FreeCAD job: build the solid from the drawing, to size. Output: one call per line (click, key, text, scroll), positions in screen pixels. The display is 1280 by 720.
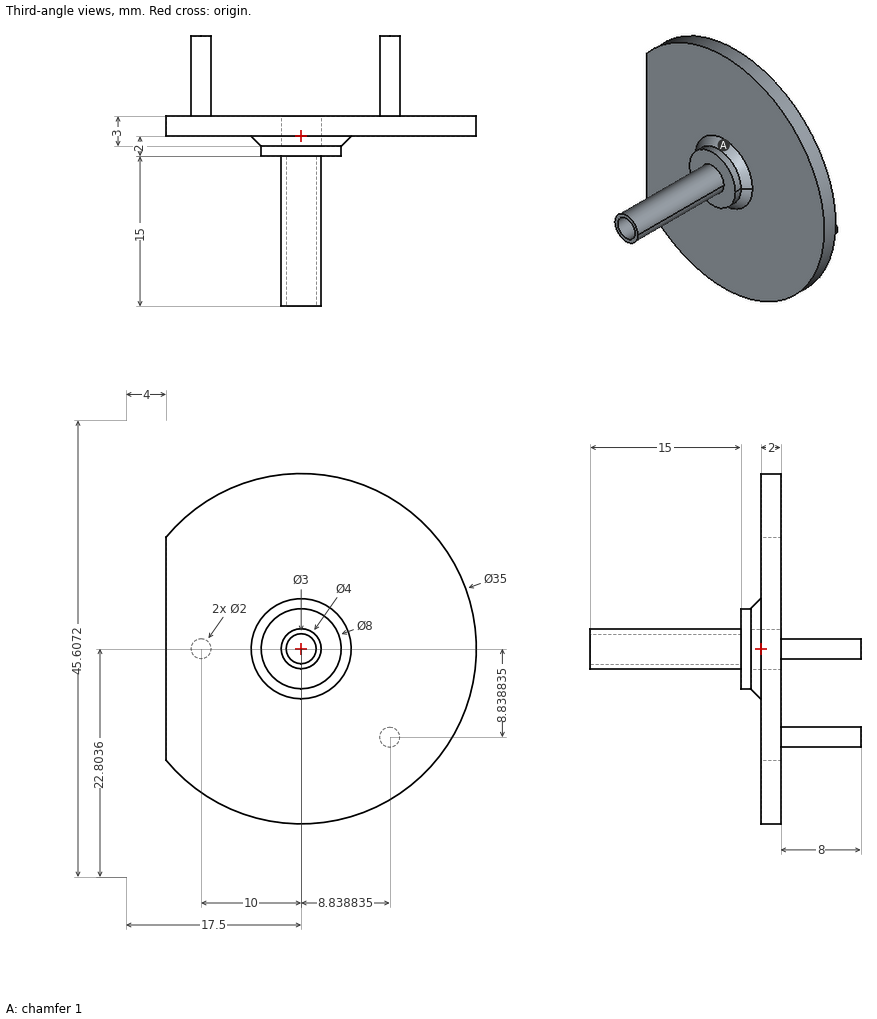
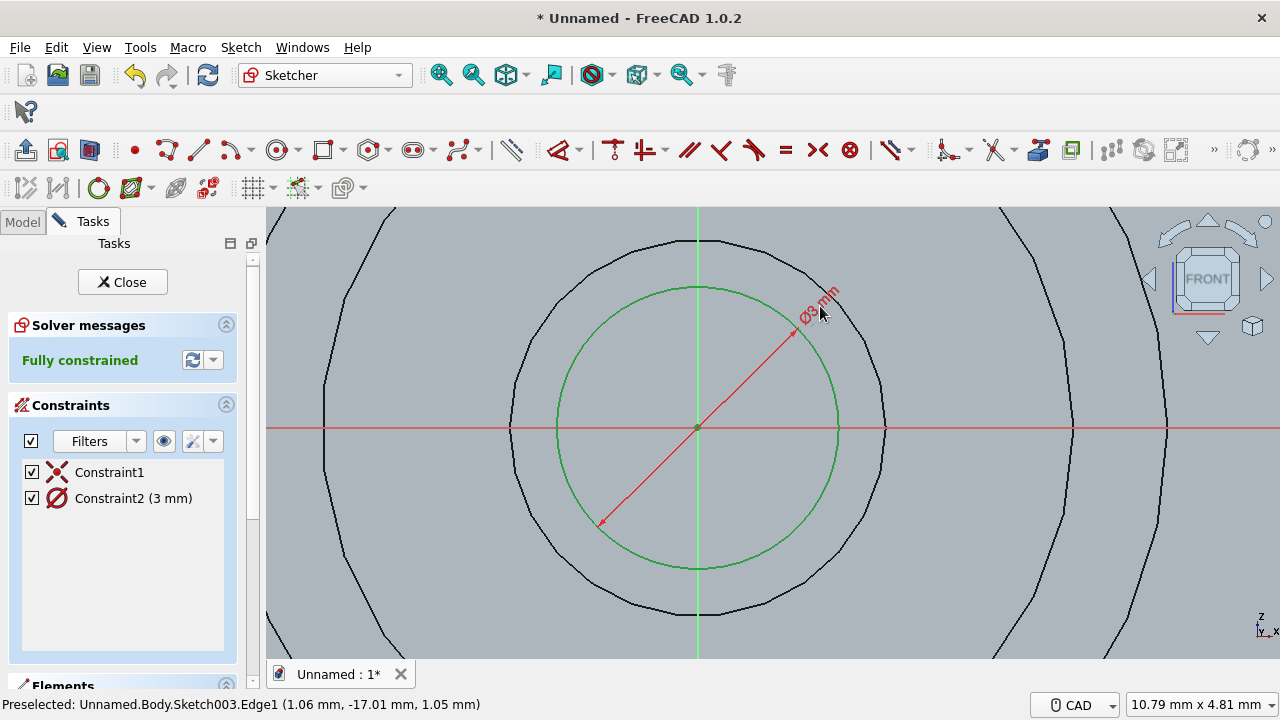
click(123, 282)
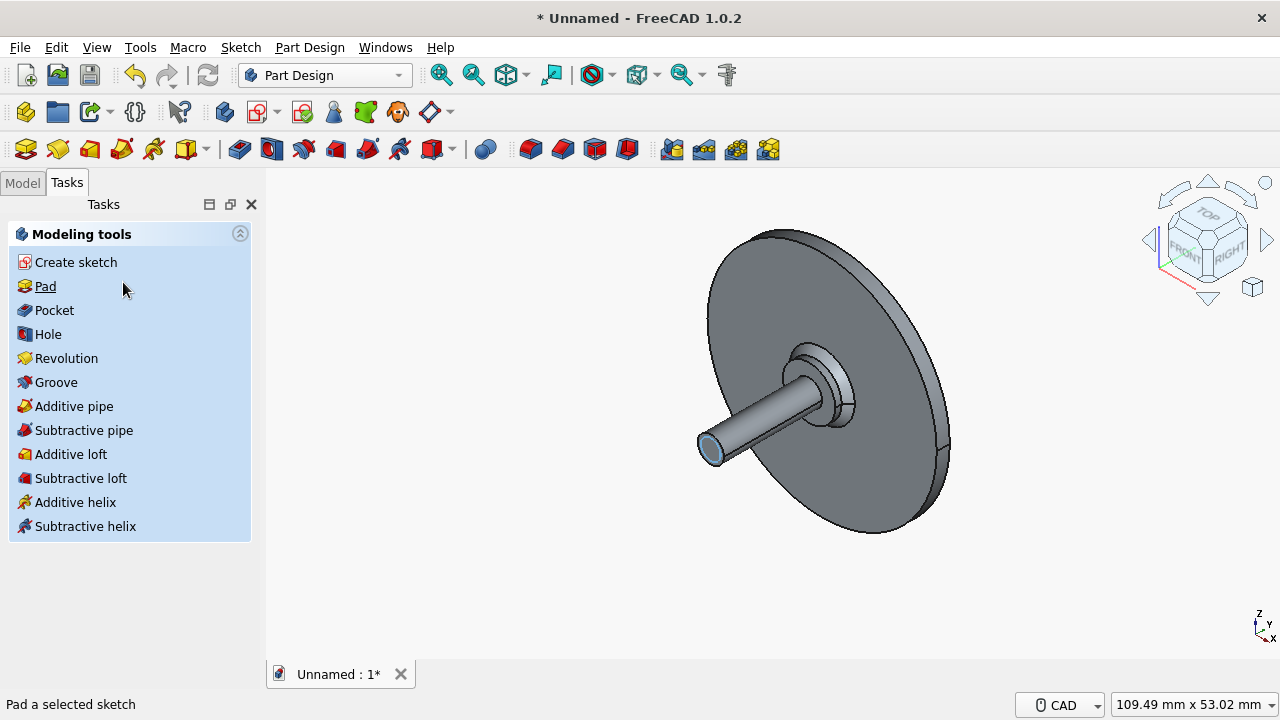
click(240, 150)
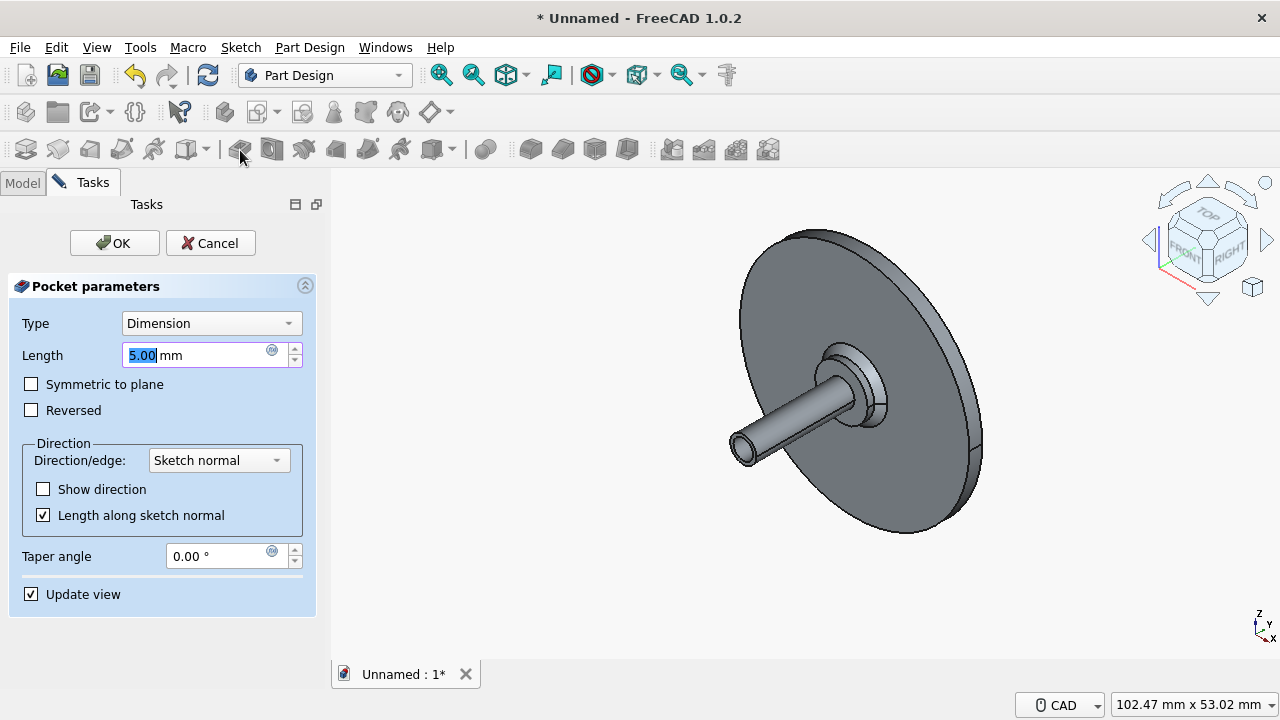
text(15)
key(Tab)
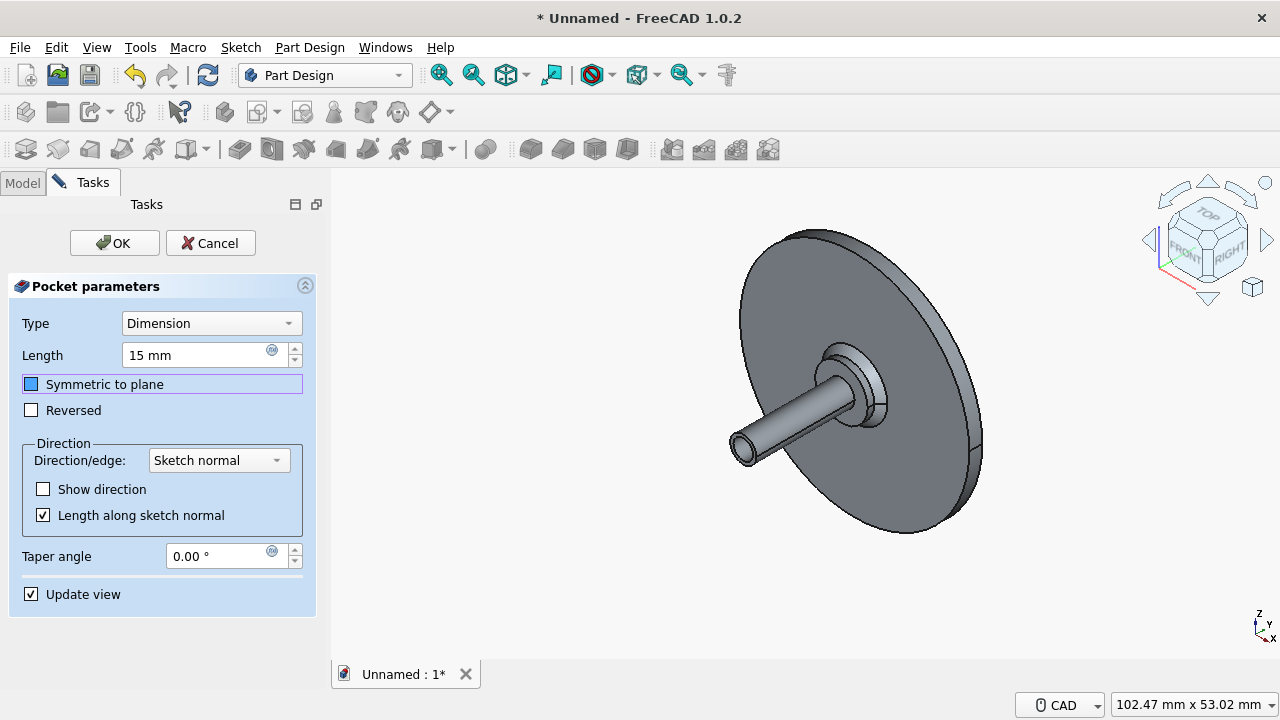
click(115, 243)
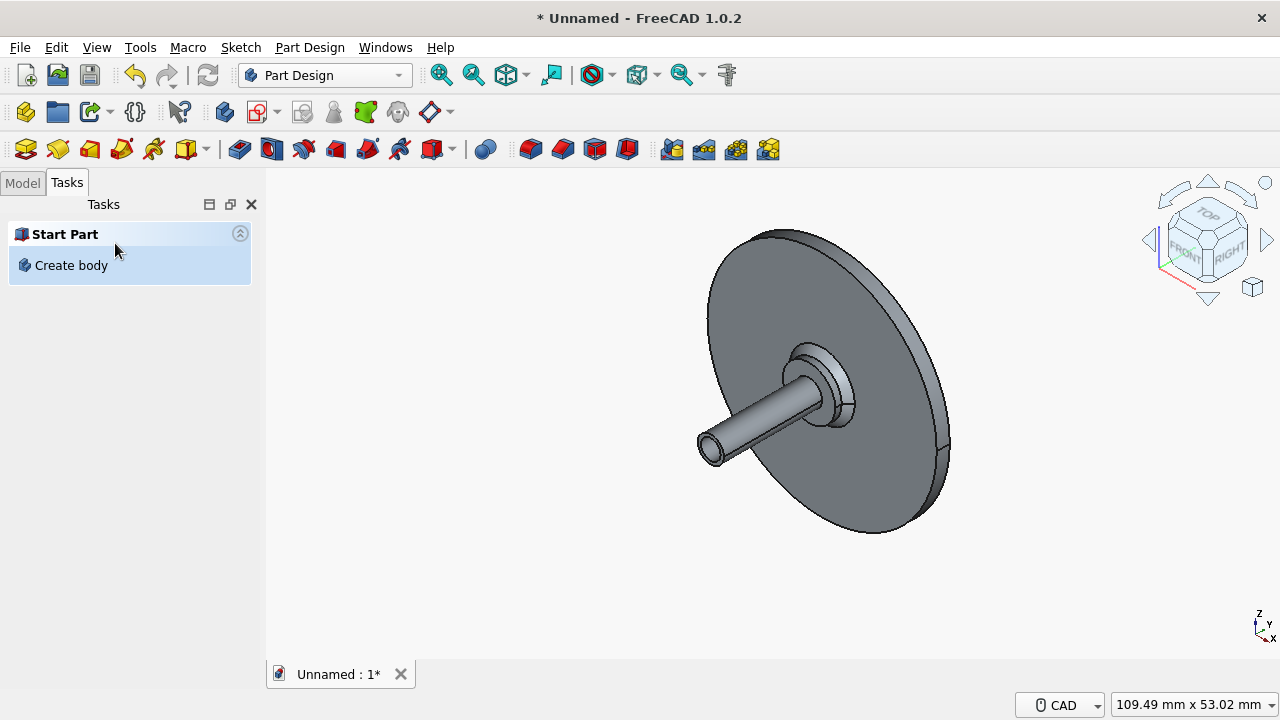
key(4)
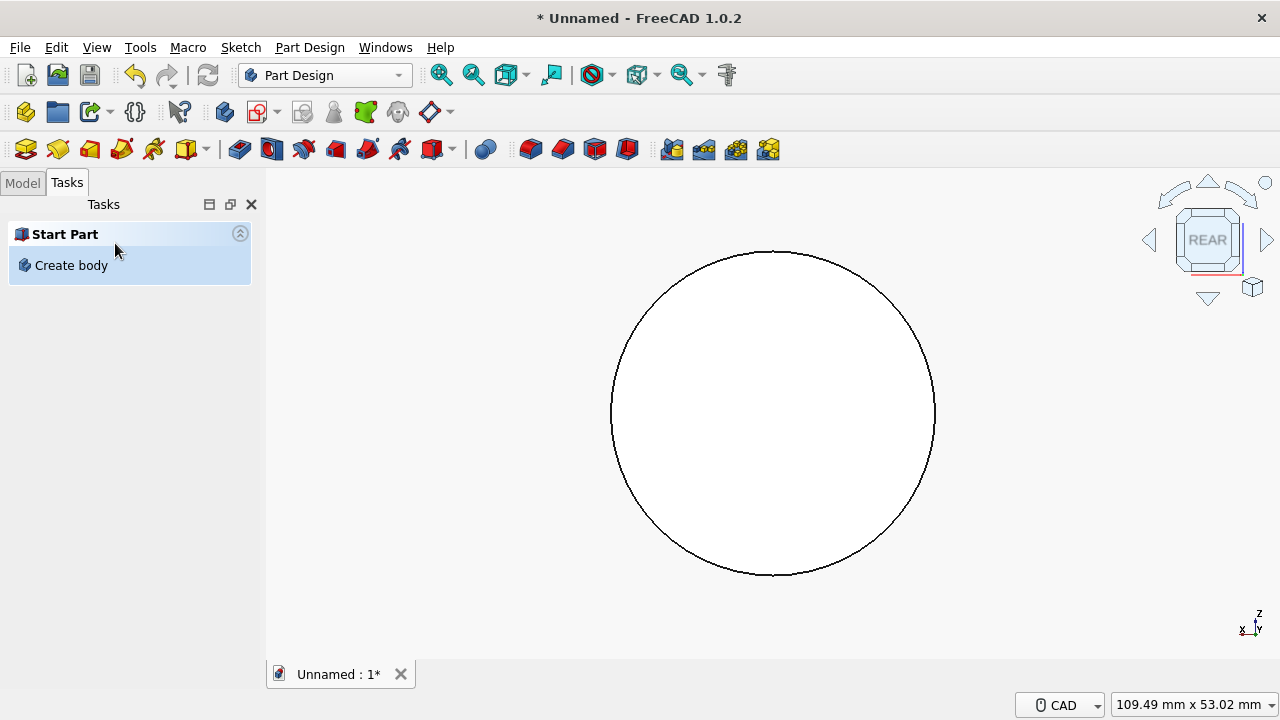
click(773, 412)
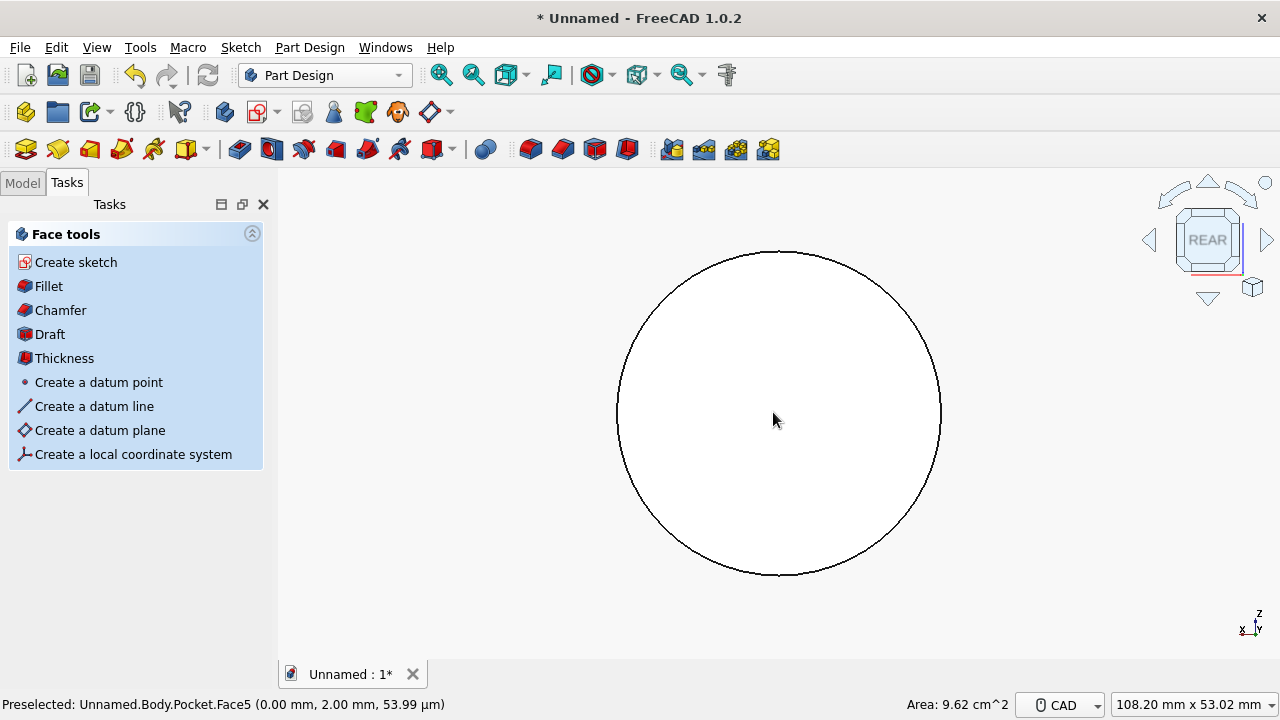
click(258, 112)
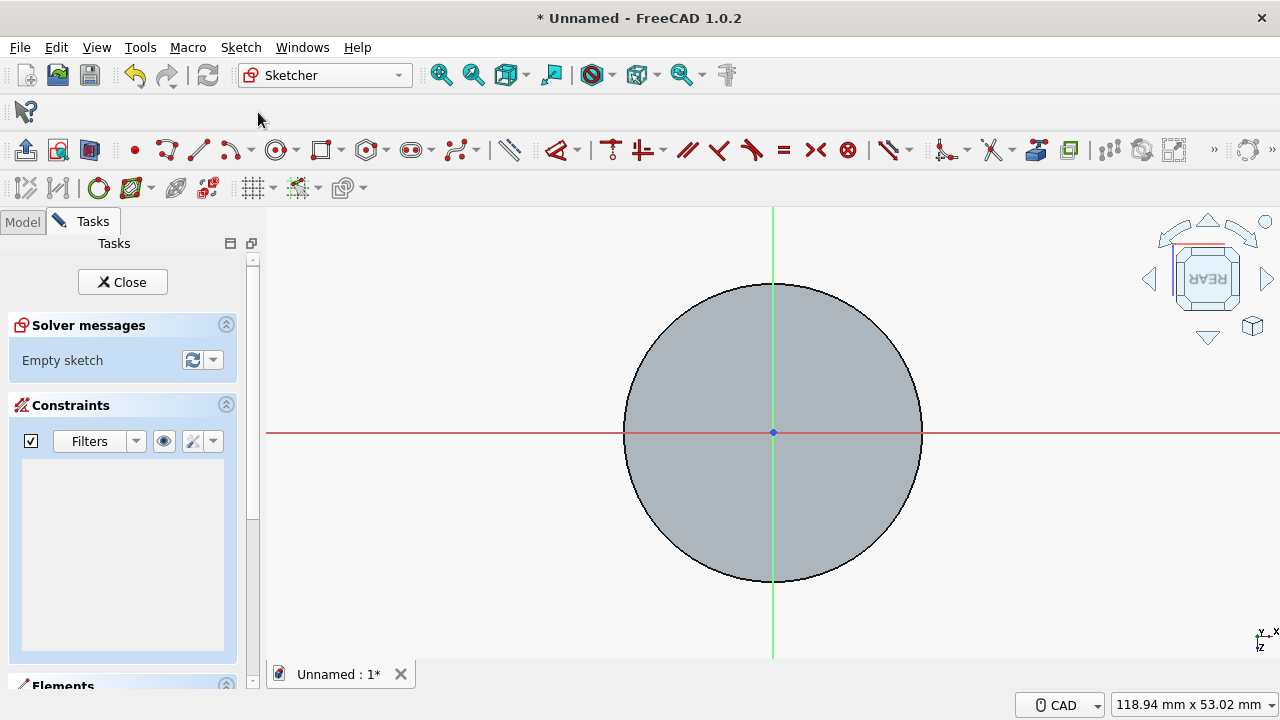
scroll(795, 379, up, 6)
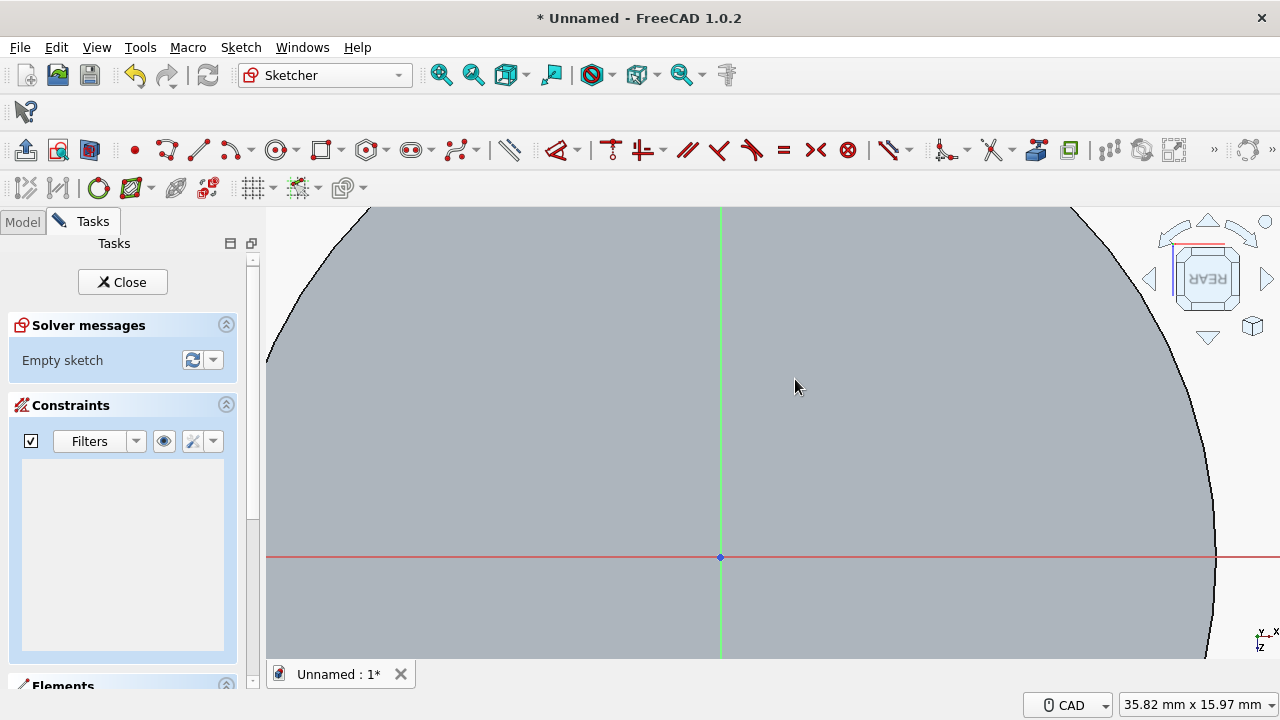
click(276, 150)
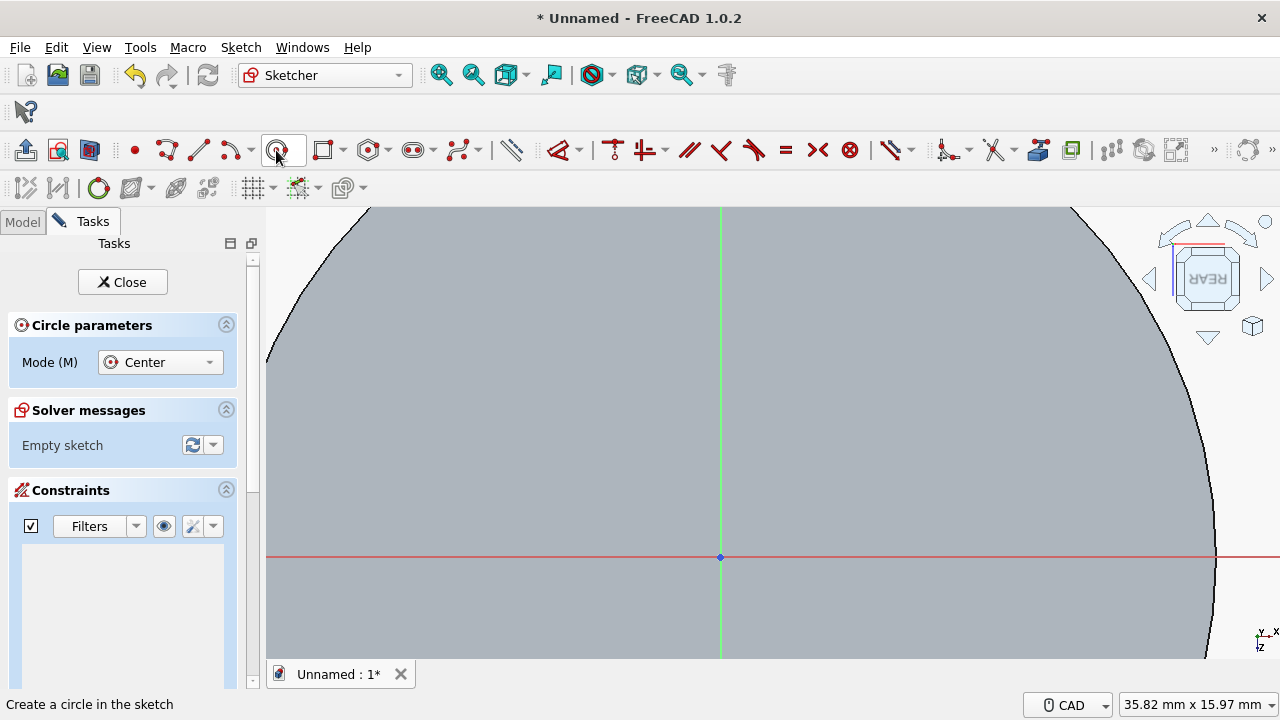
click(438, 557)
click(458, 537)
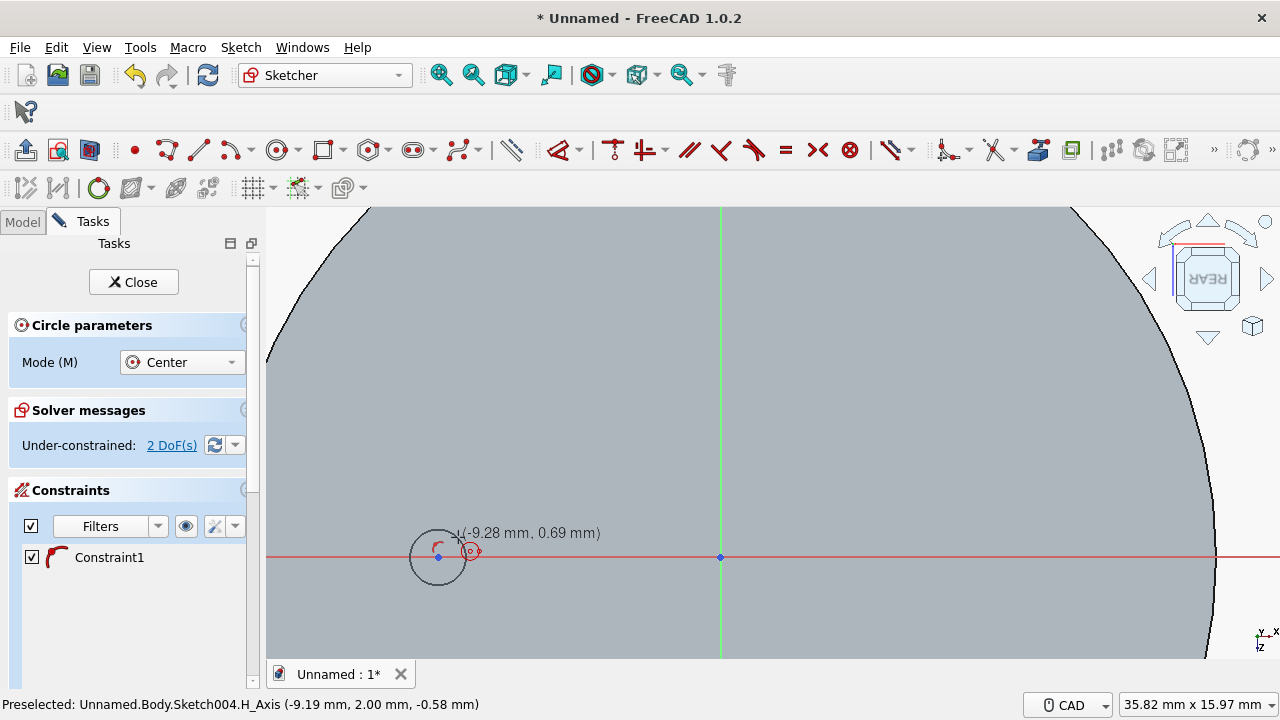
click(971, 307)
click(991, 287)
key(Escape)